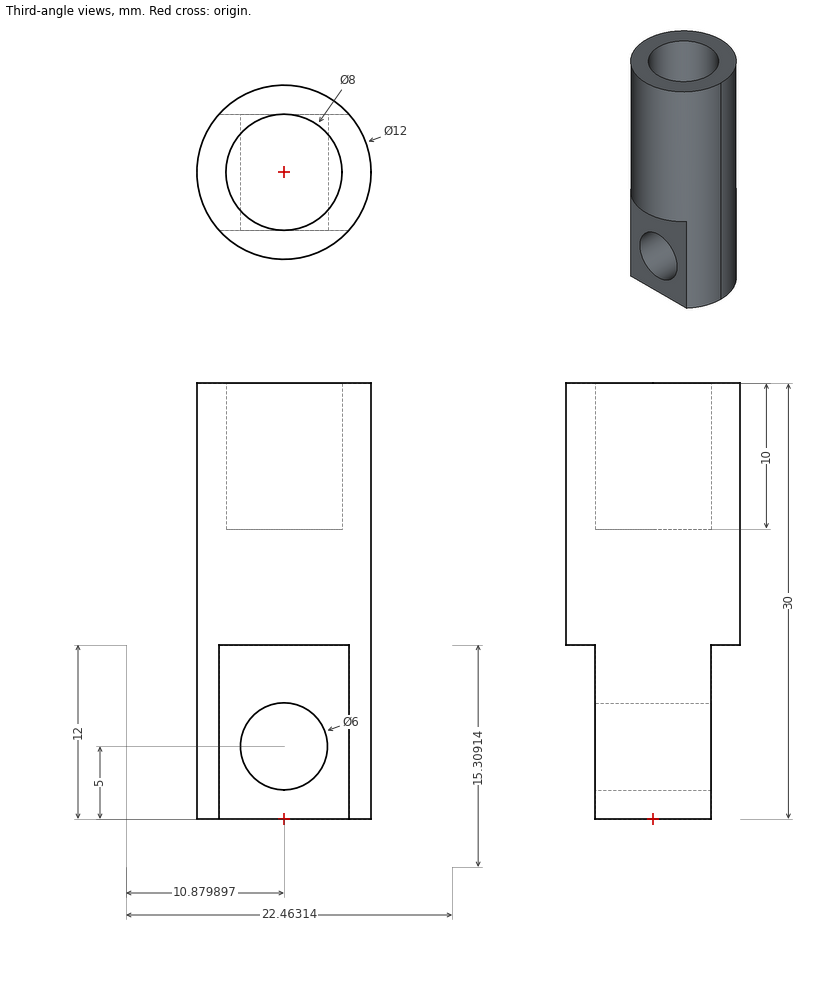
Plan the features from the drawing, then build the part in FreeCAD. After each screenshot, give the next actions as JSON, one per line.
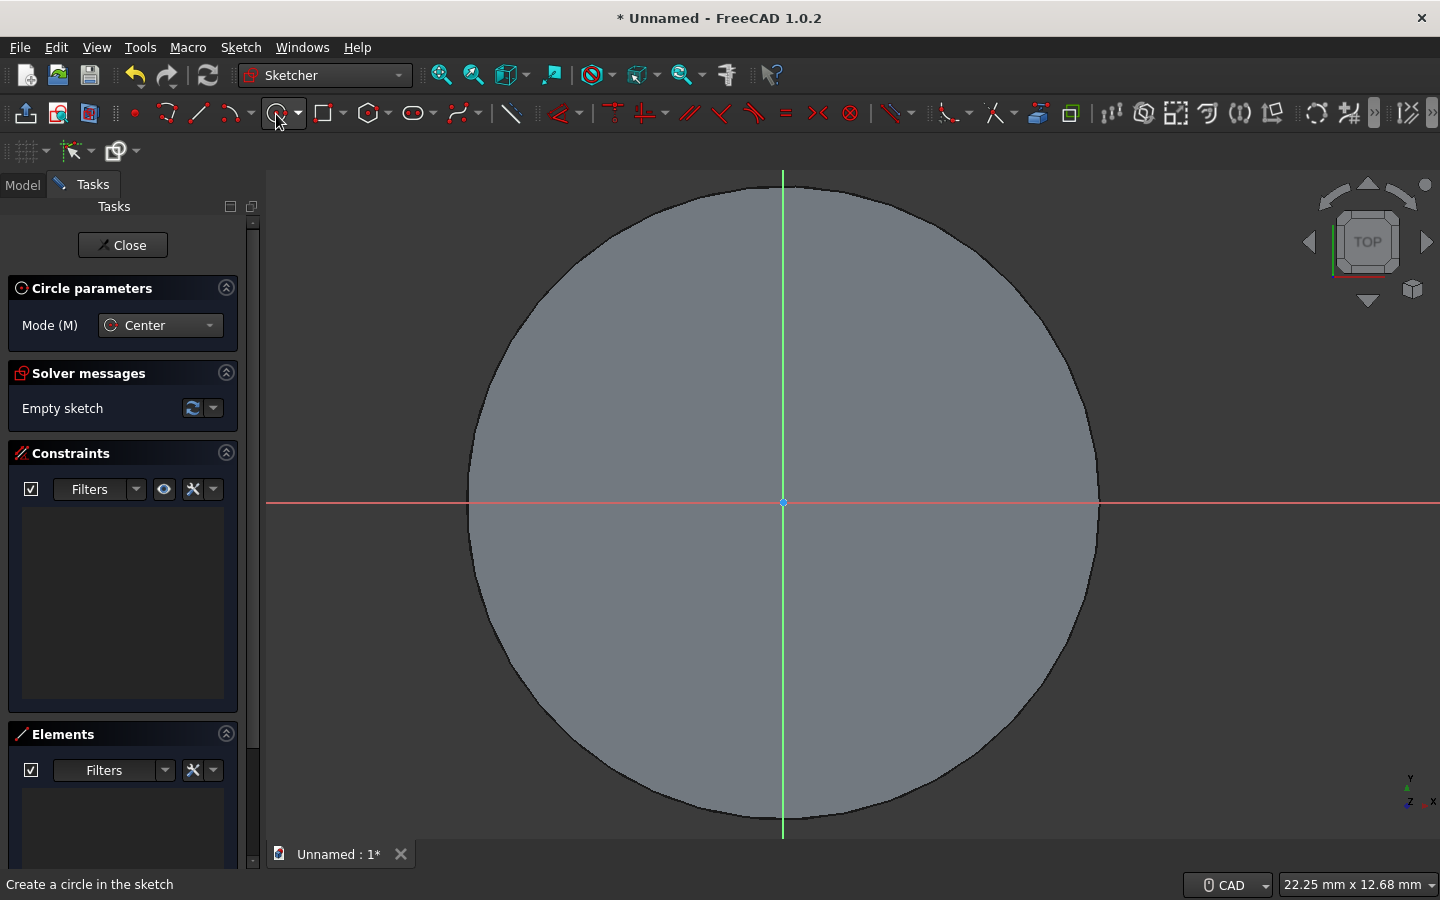
{"action": "left_click", "coordinate": [783, 503]}
{"action": "mouse_move", "coordinate": [932, 354]}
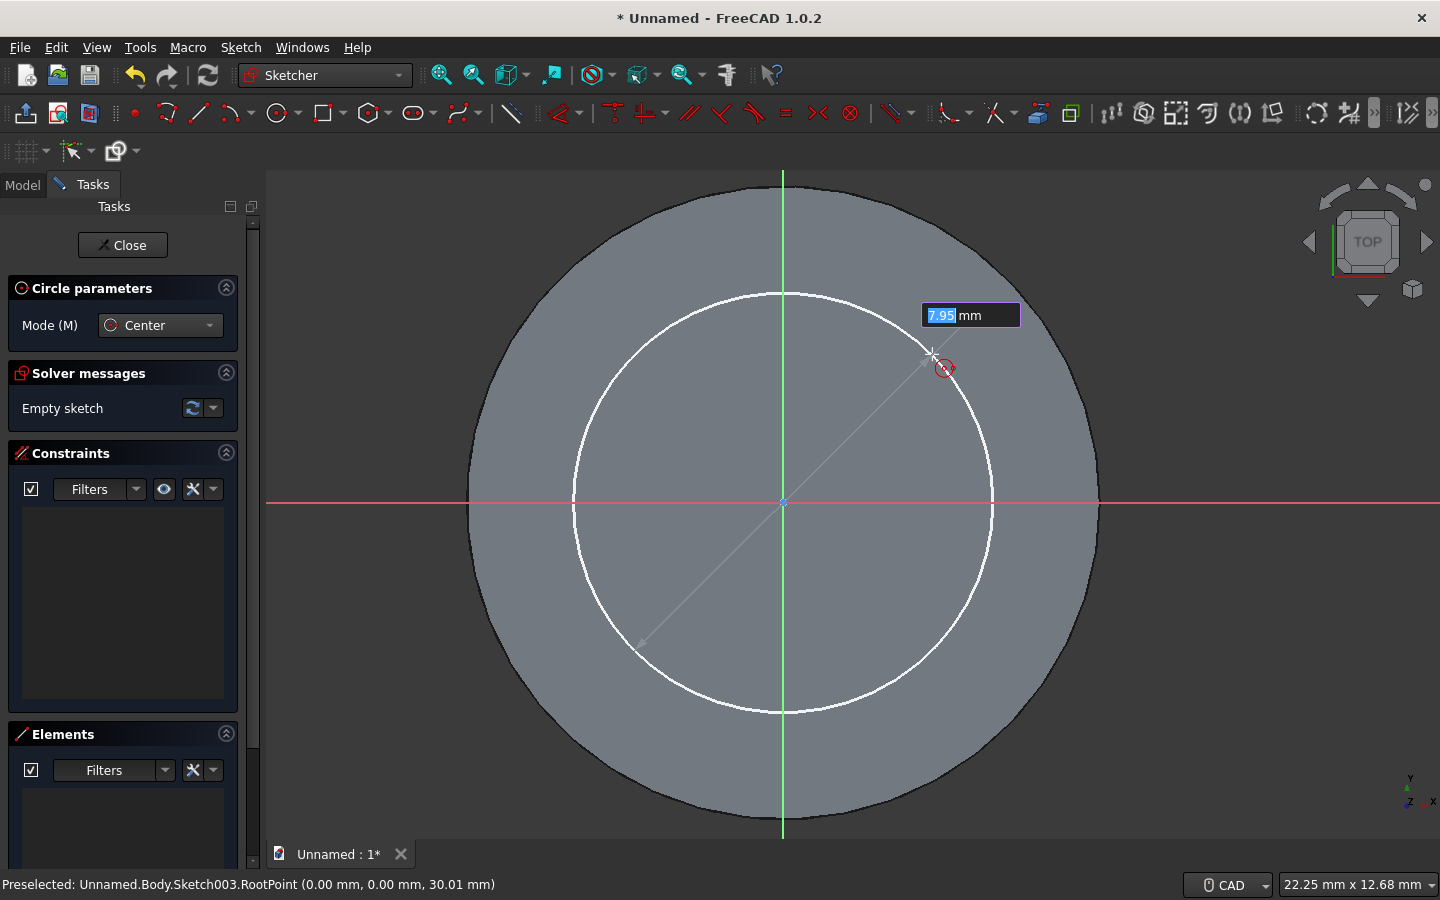
{"action": "type", "text": "8"}
{"action": "key", "text": "Return"}
{"action": "key", "text": "Escape"}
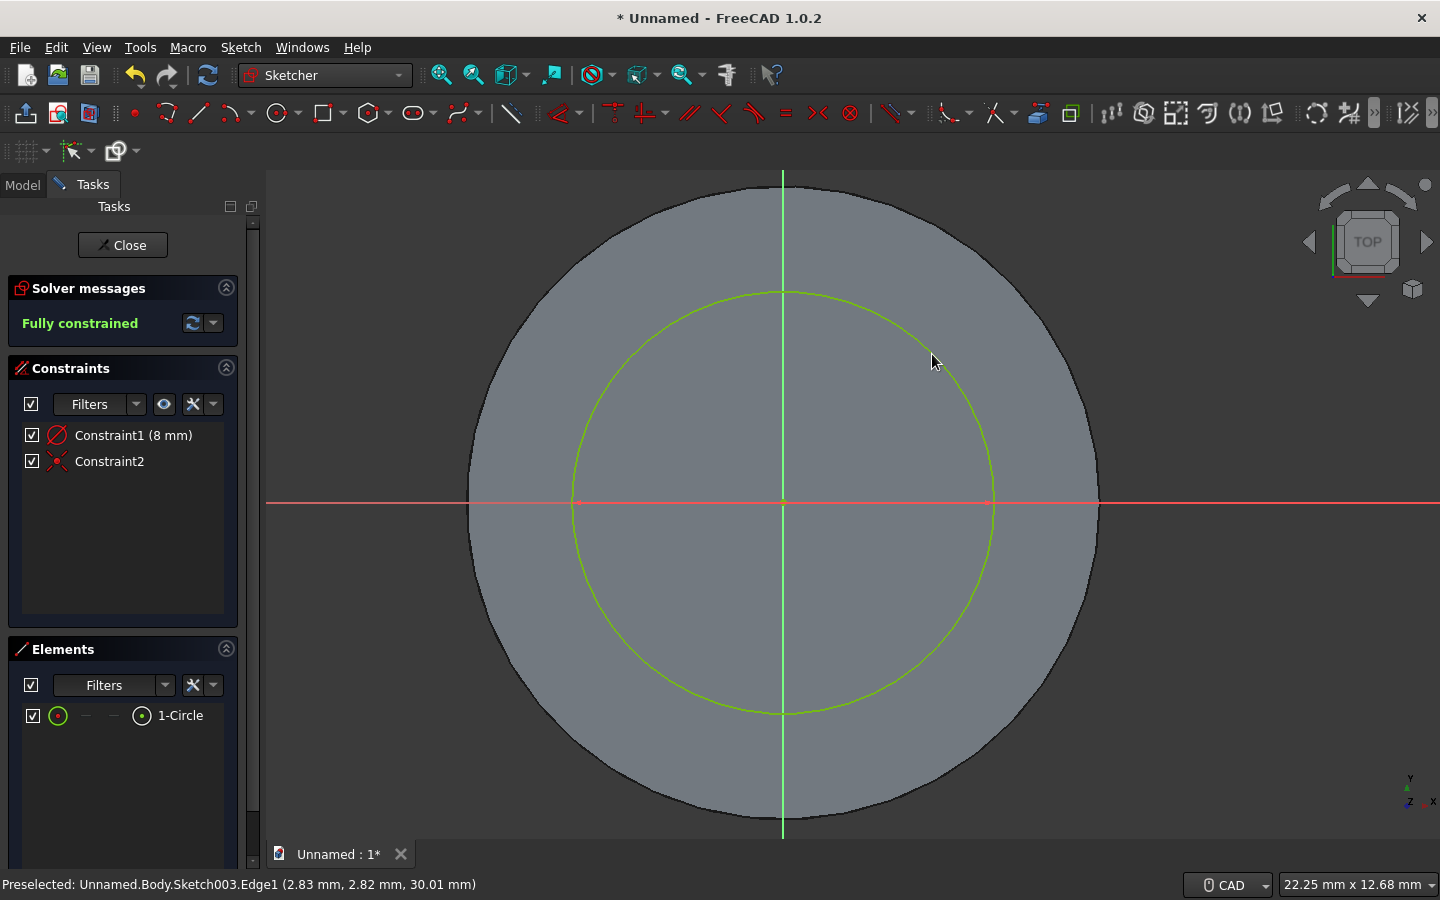
{"action": "left_click", "coordinate": [123, 245]}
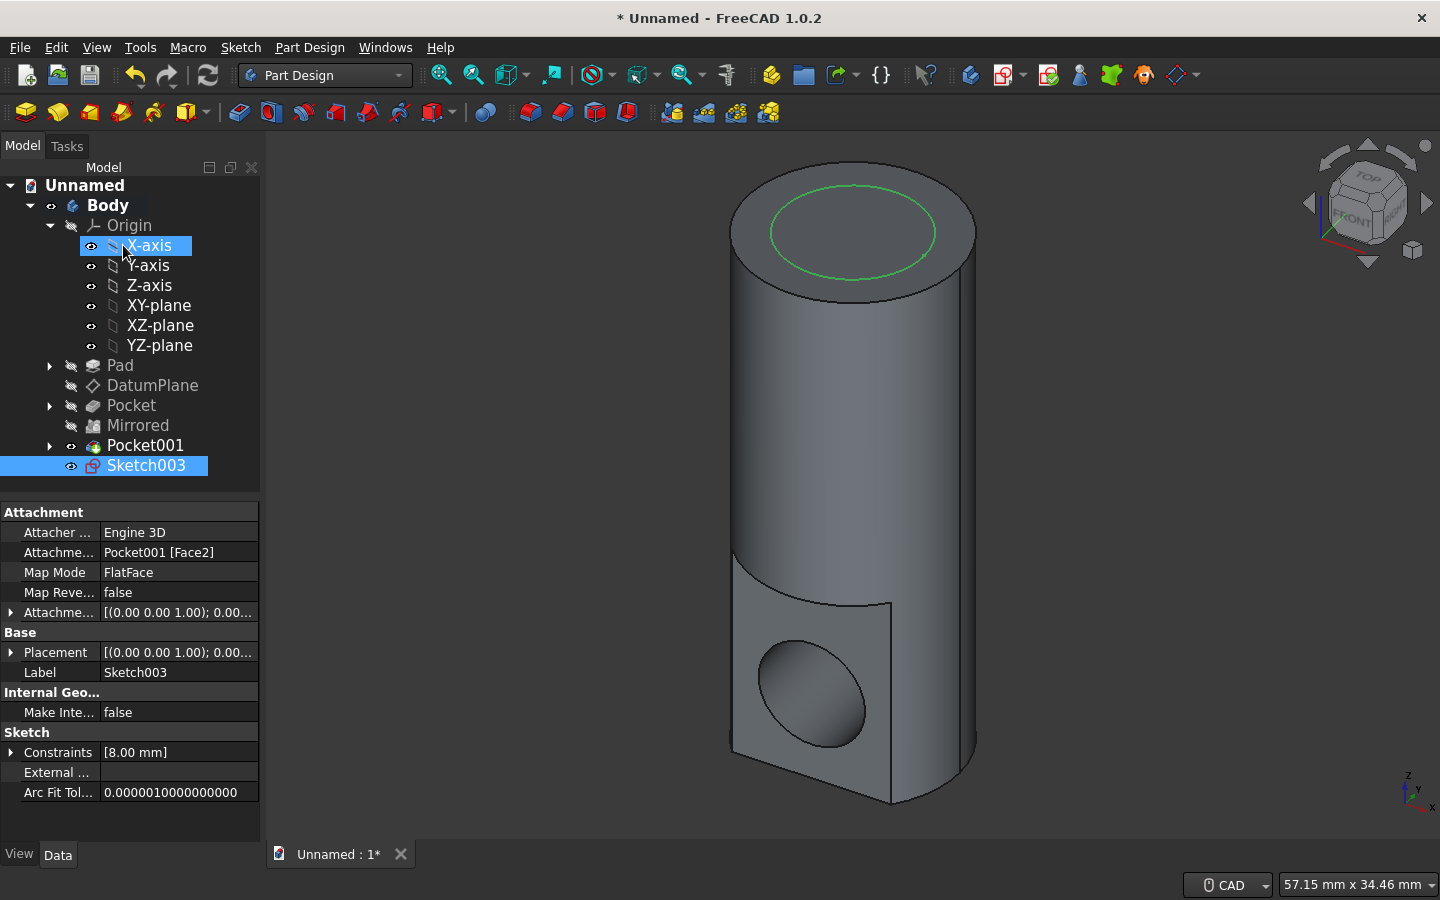
{"action": "left_click", "coordinate": [240, 112]}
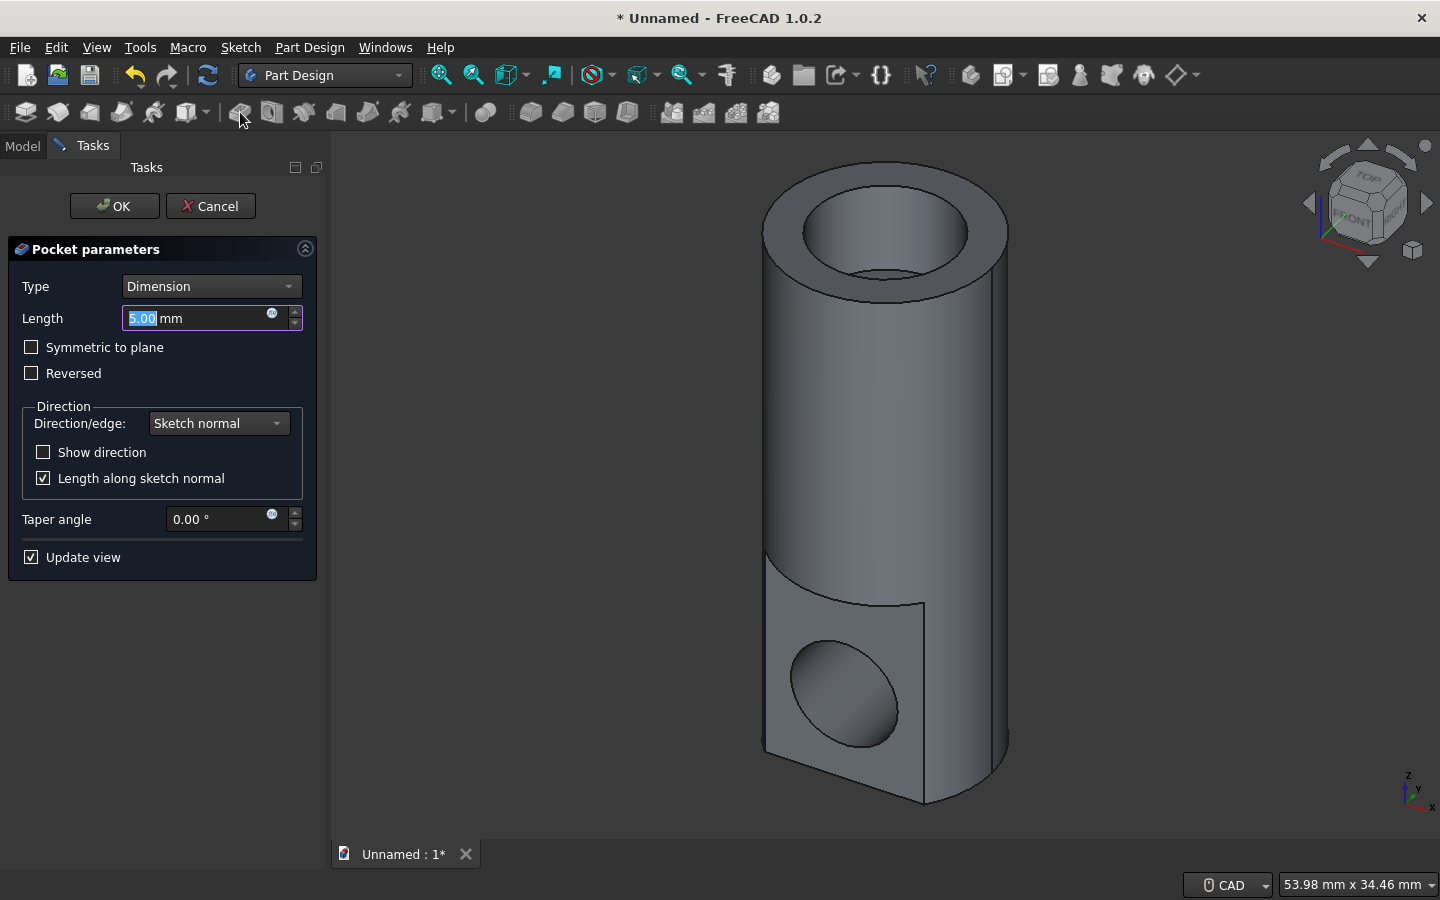
{"action": "type", "text": "10"}
{"action": "key", "text": "Tab"}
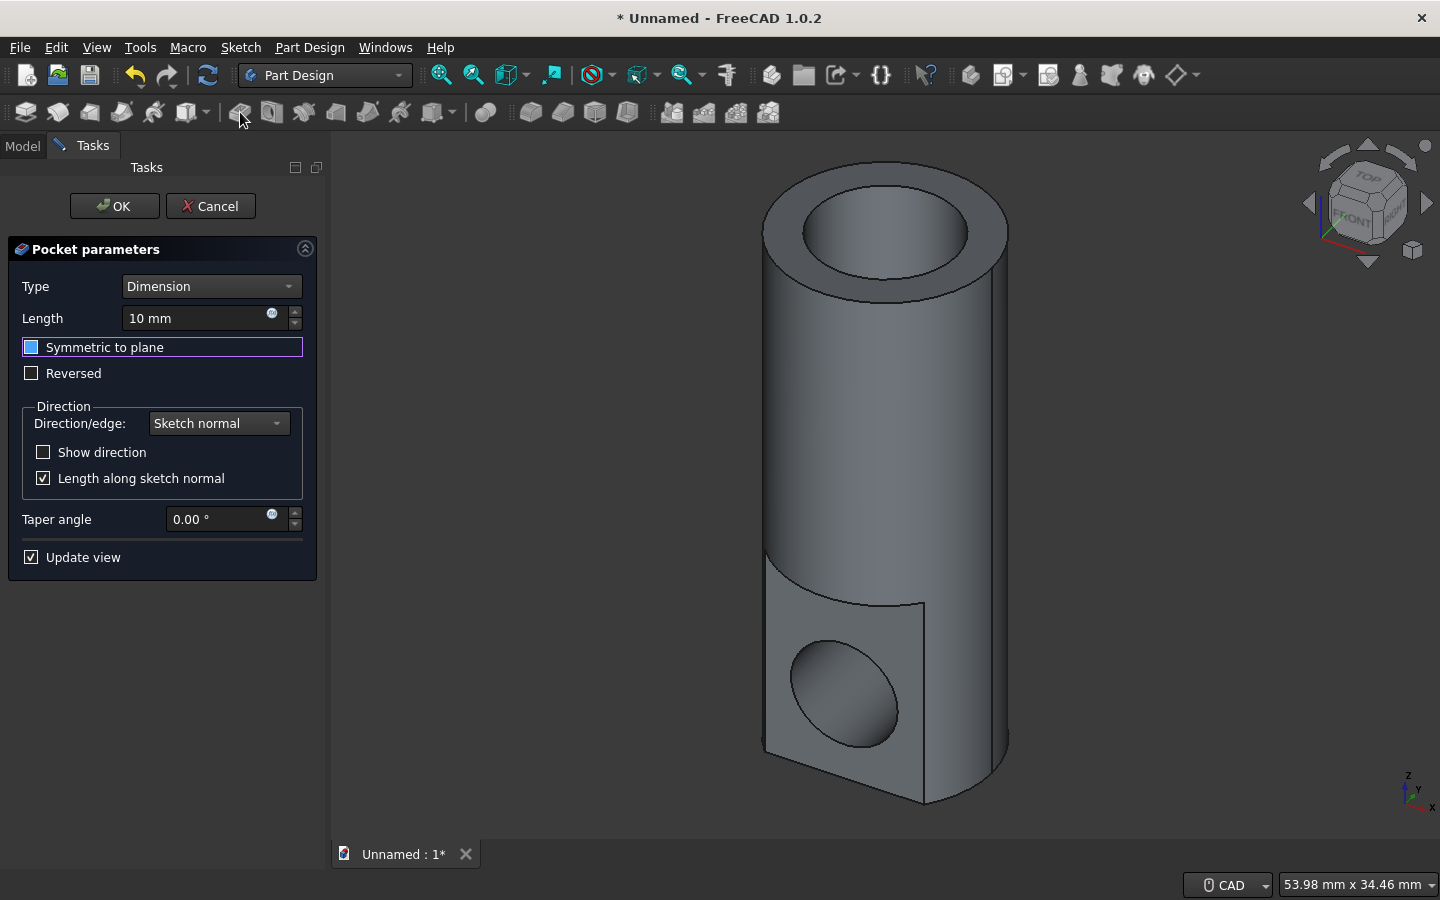
{"action": "left_click", "coordinate": [115, 206]}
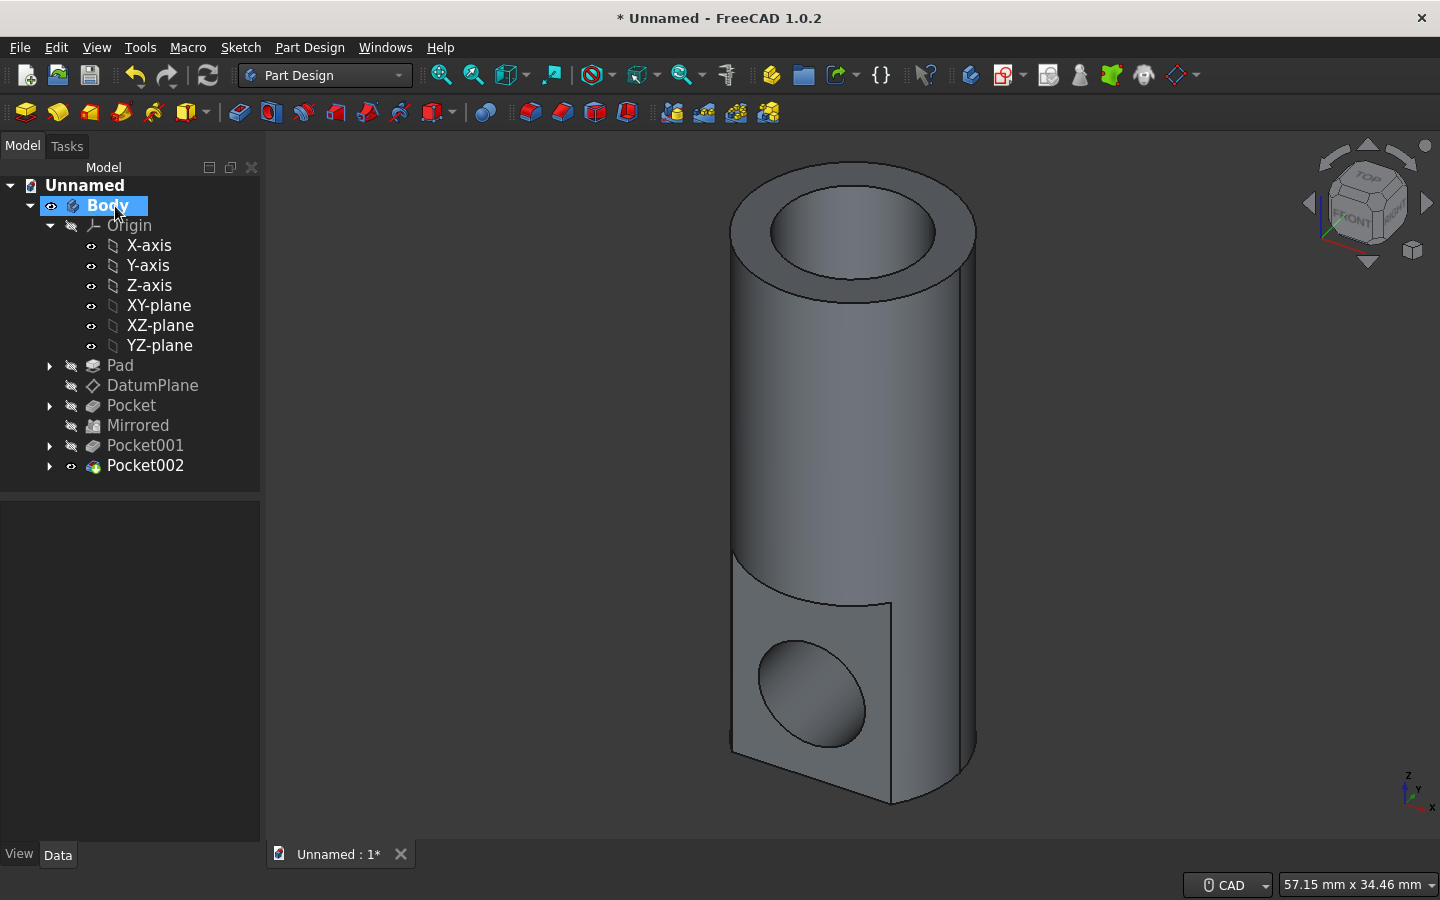
{"action": "key", "text": "0"}